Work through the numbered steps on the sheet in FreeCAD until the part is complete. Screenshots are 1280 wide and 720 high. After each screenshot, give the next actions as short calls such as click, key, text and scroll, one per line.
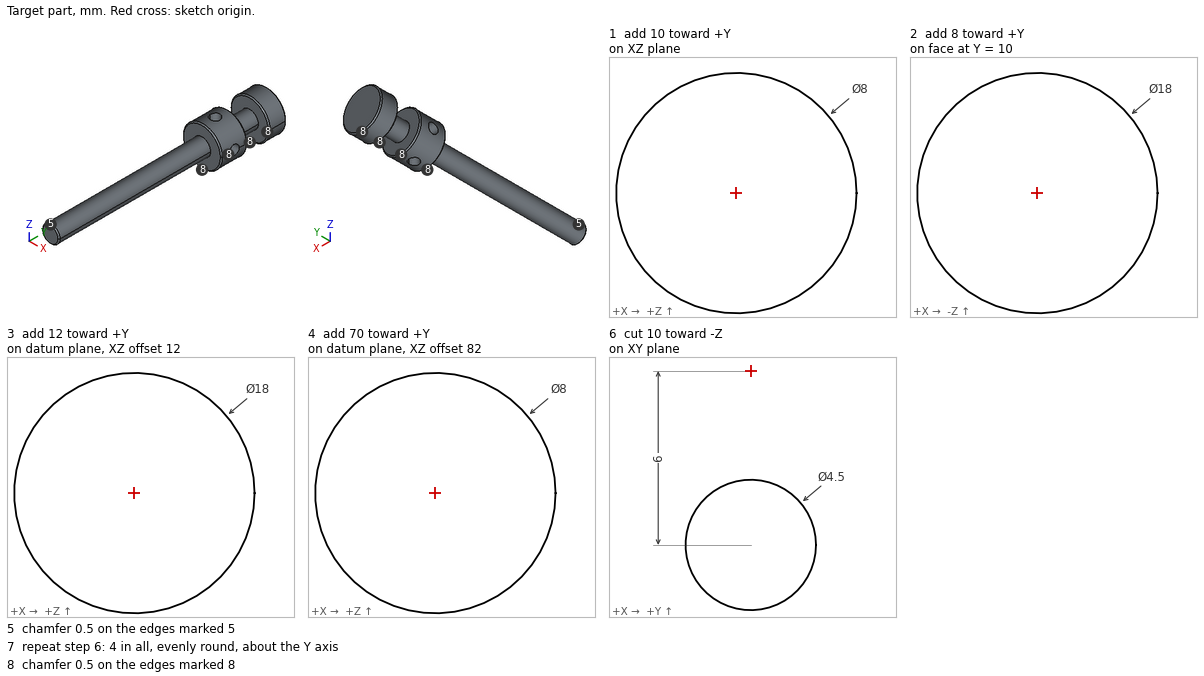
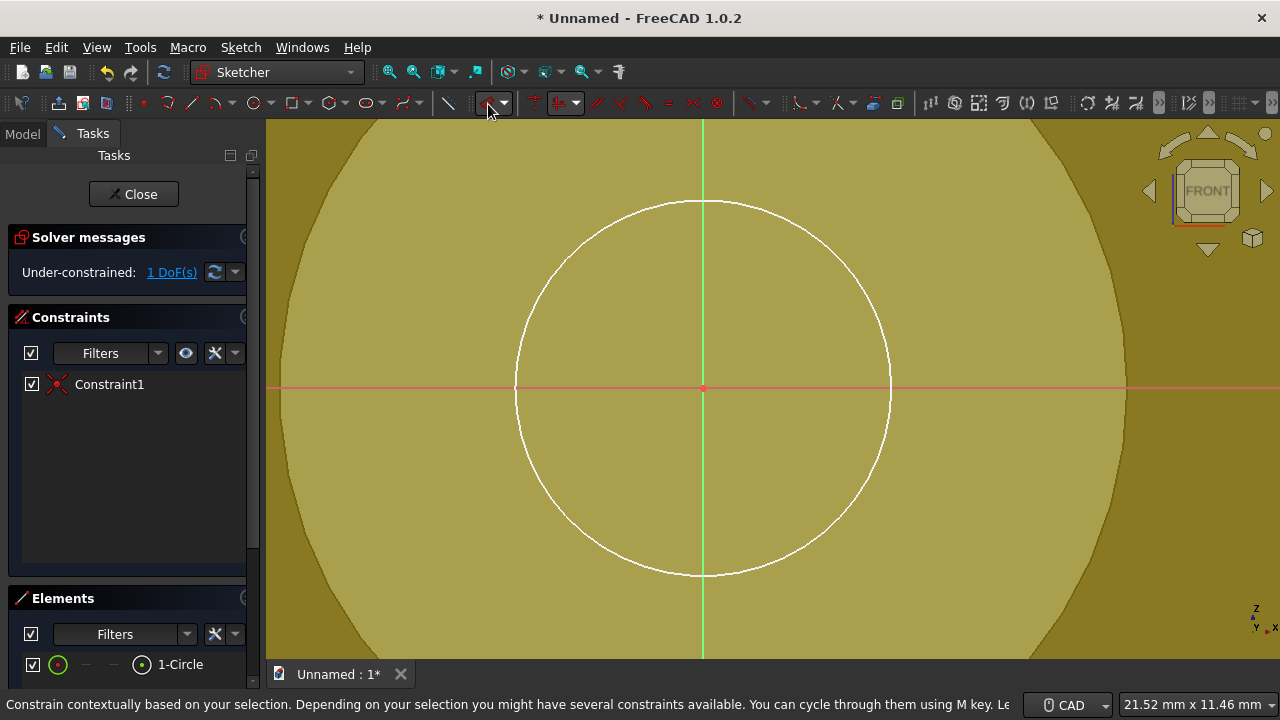
click(836, 255)
click(859, 232)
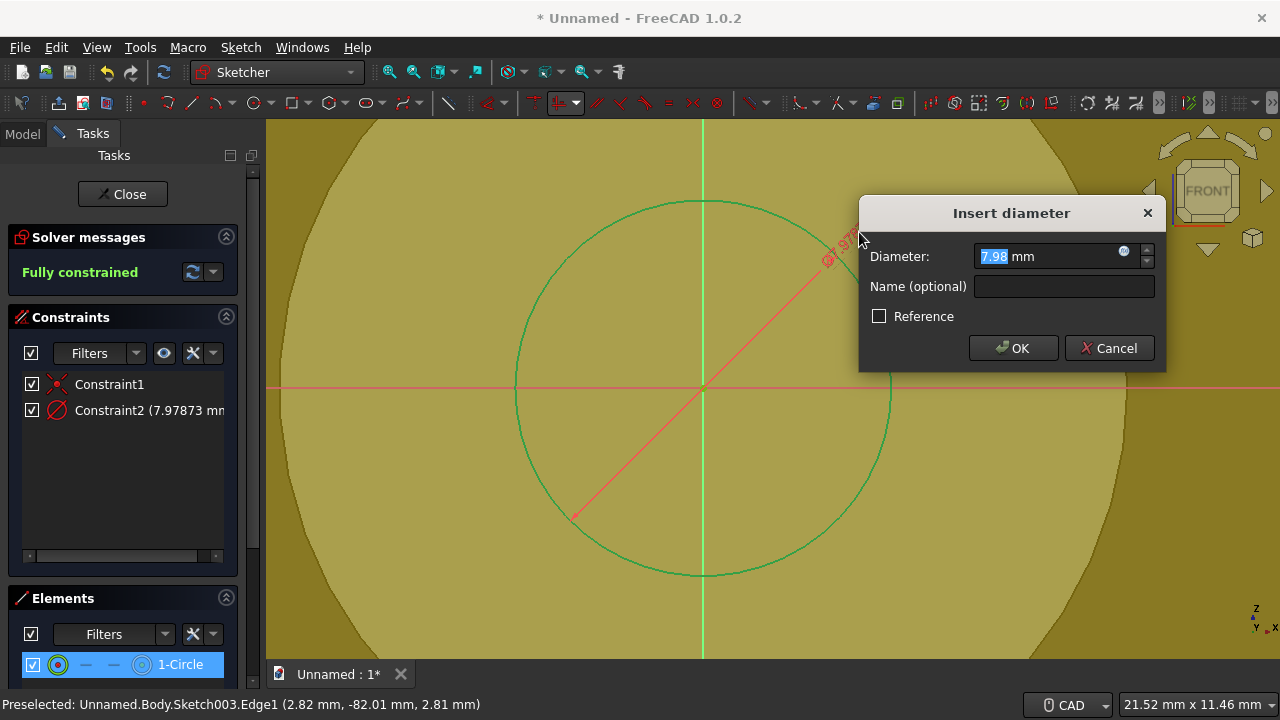
text(8)
key(Return)
key(Escape)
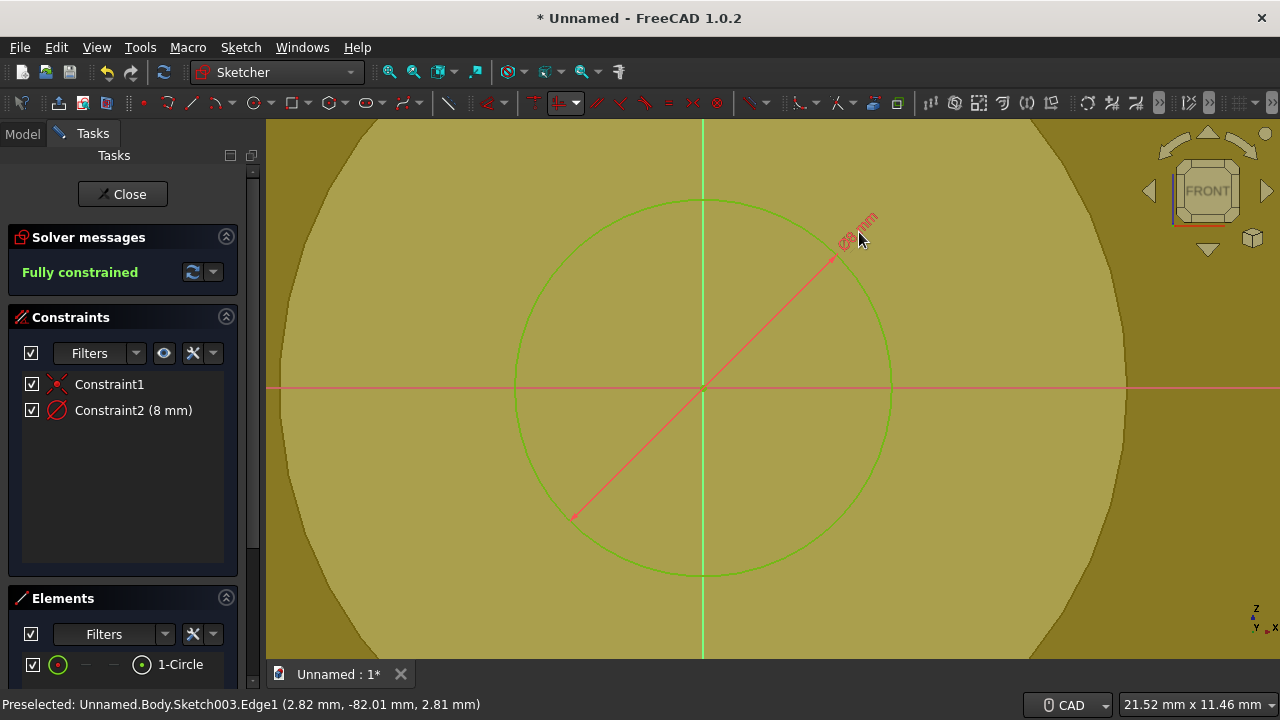
click(123, 194)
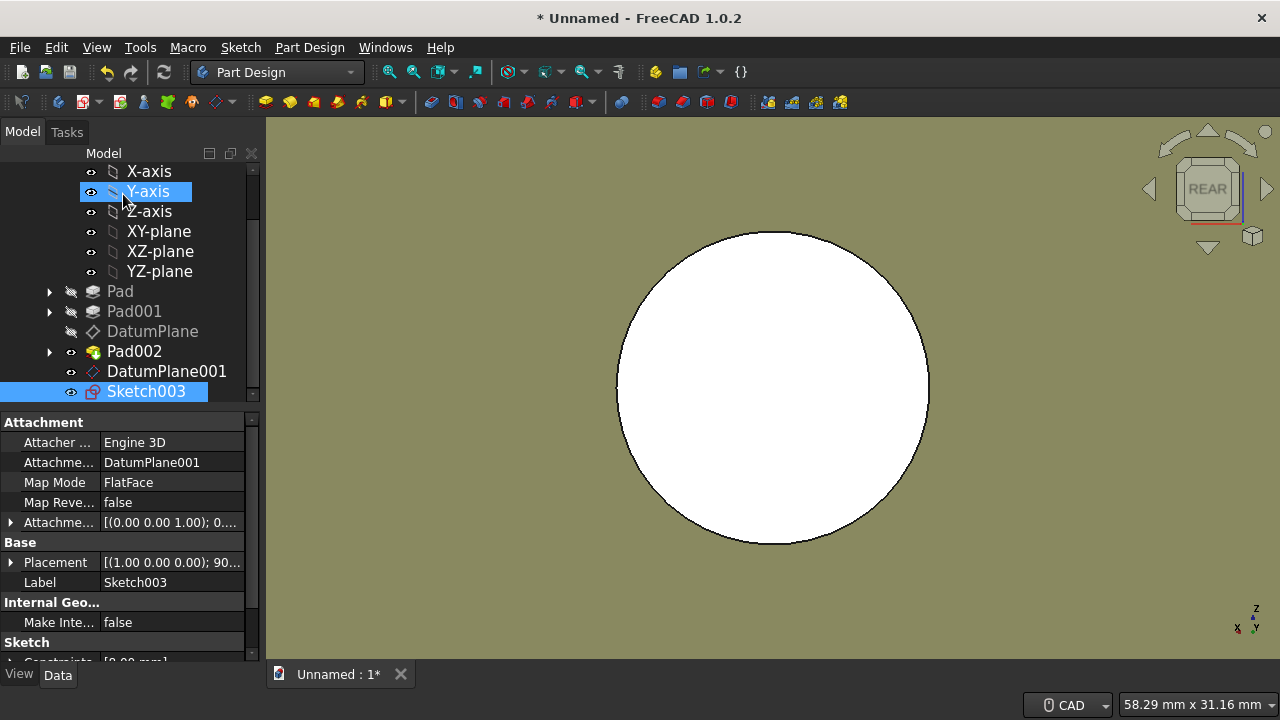
click(266, 102)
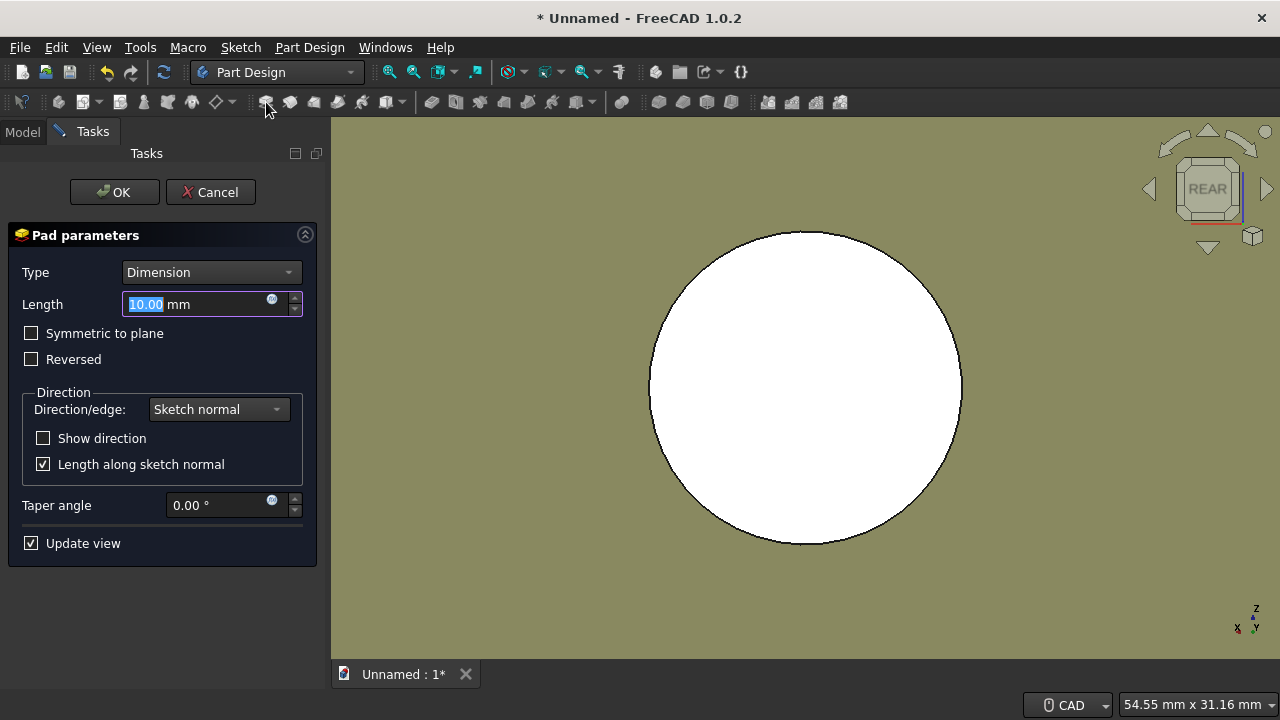
text(70)
key(Tab)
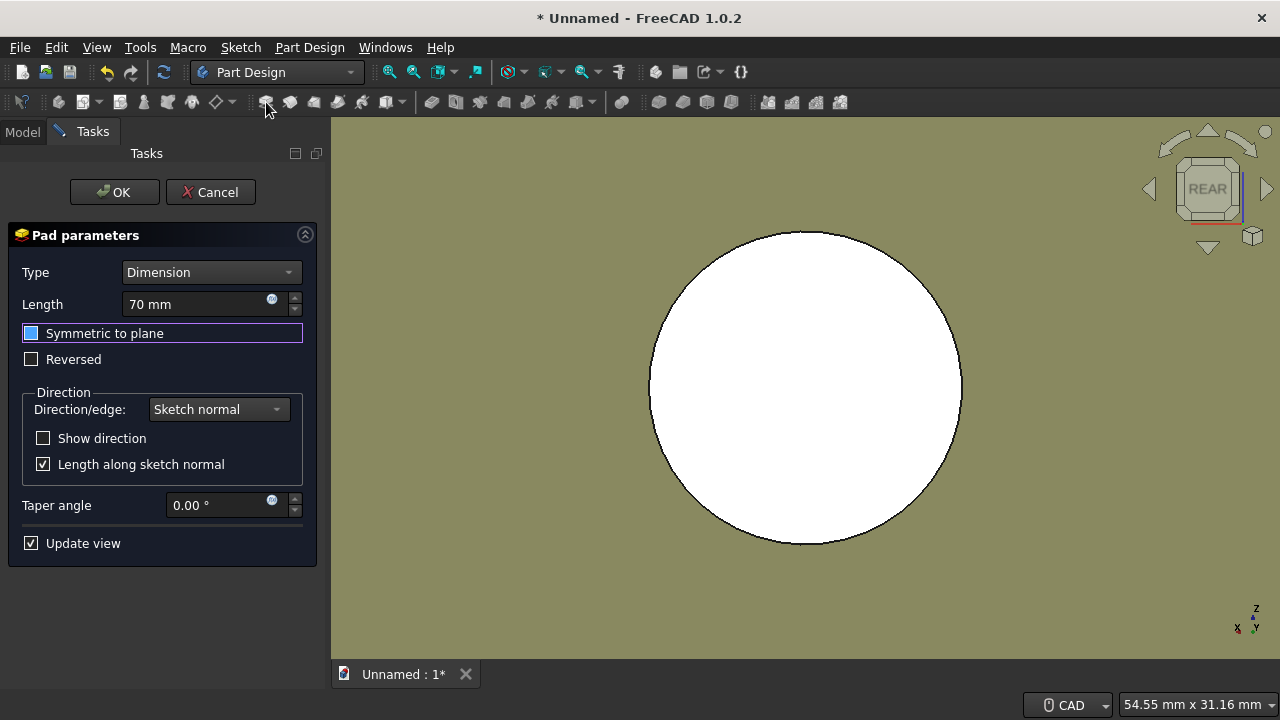
click(30, 359)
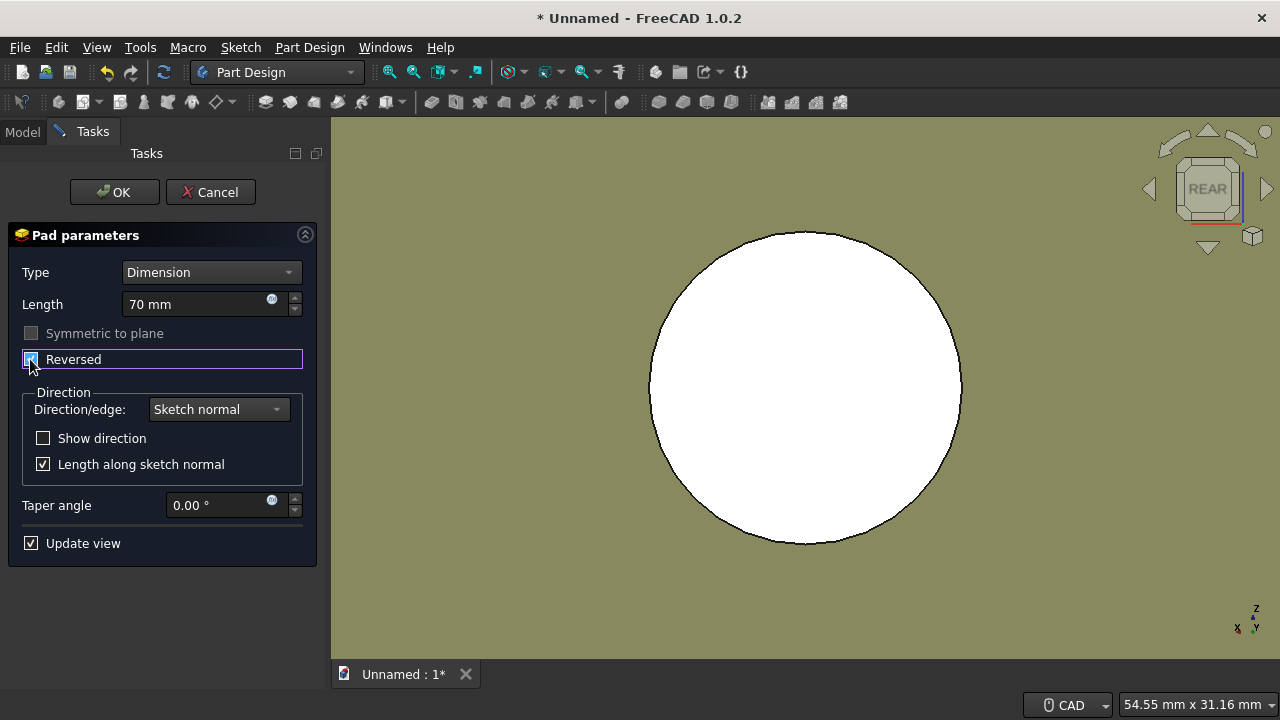
click(115, 192)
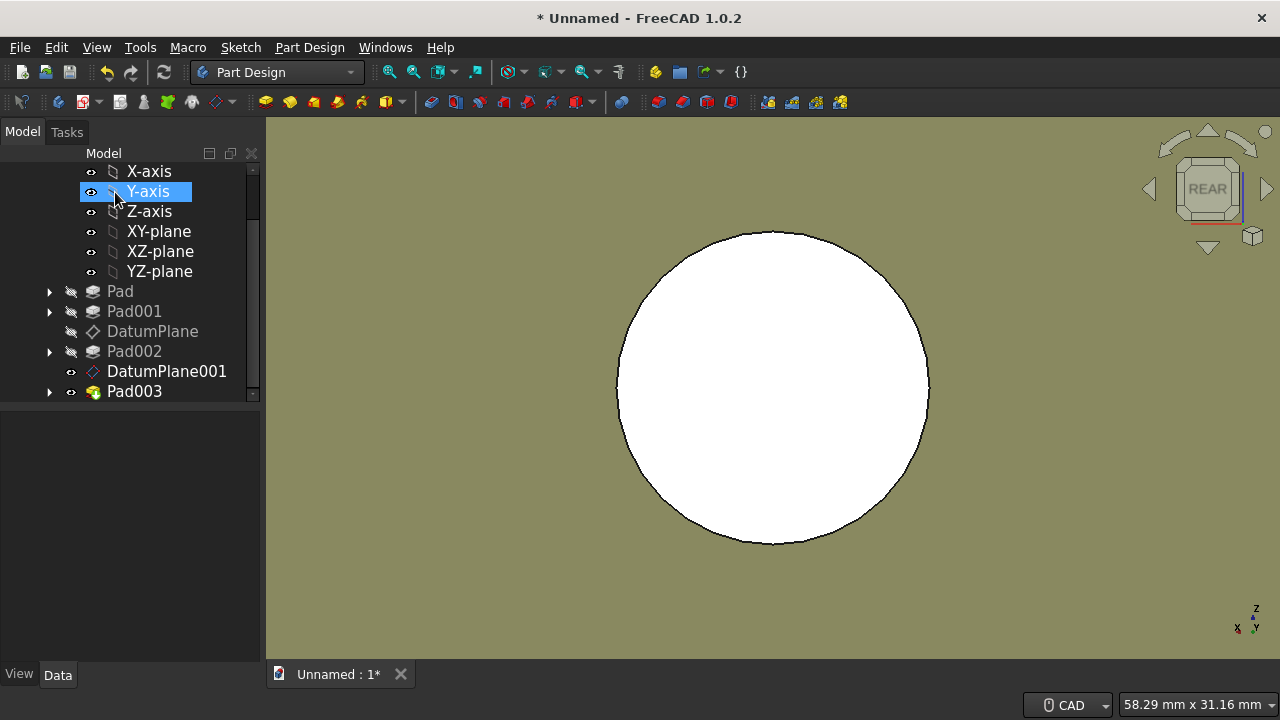
click(116, 372)
key(space)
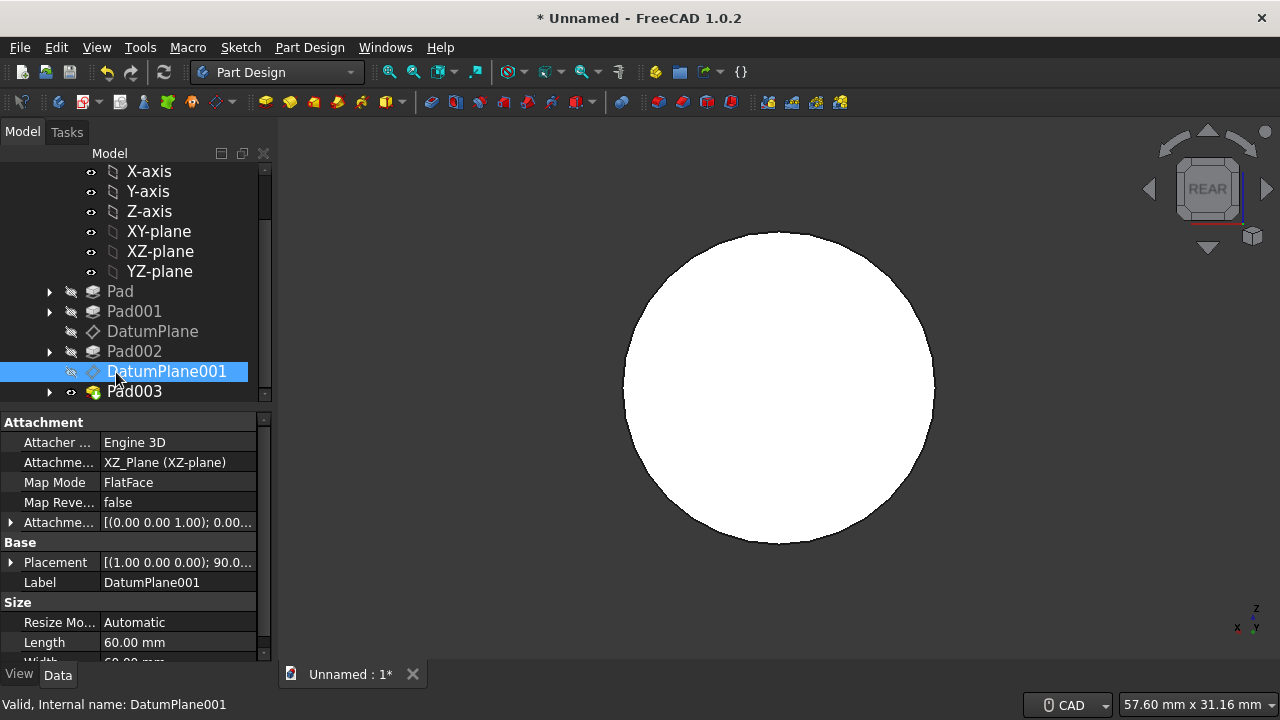
key(0)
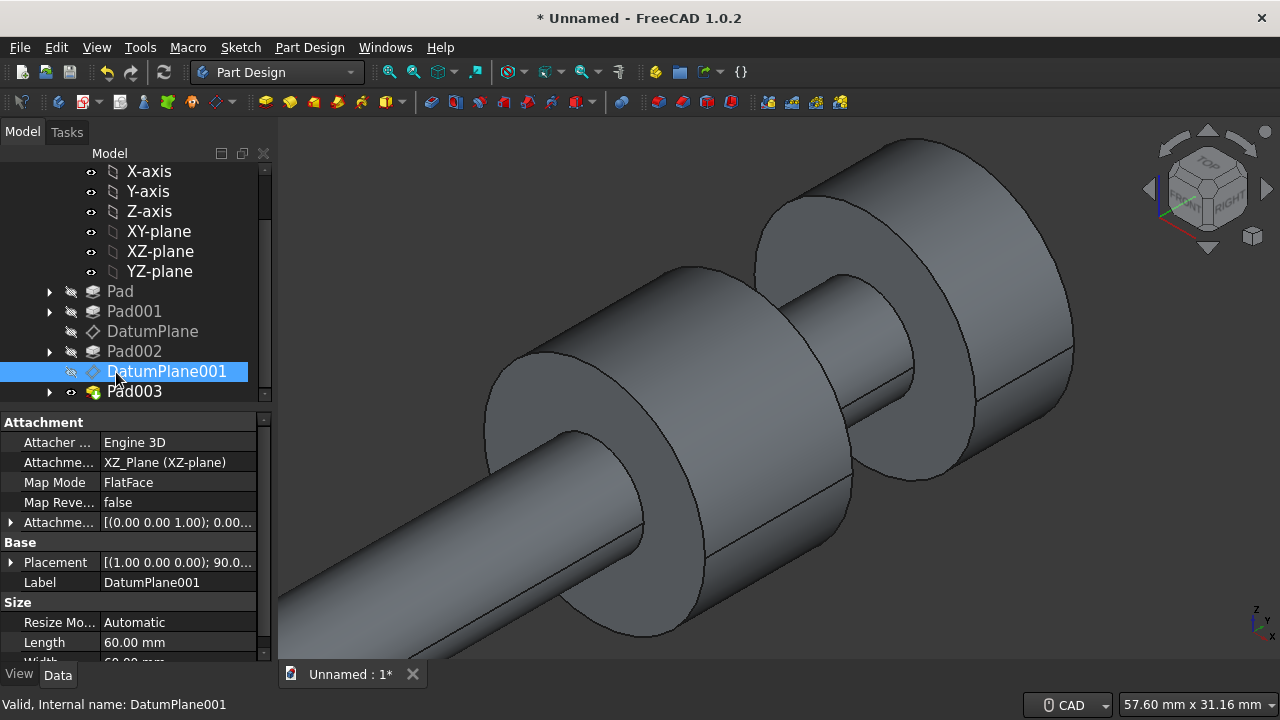
click(390, 72)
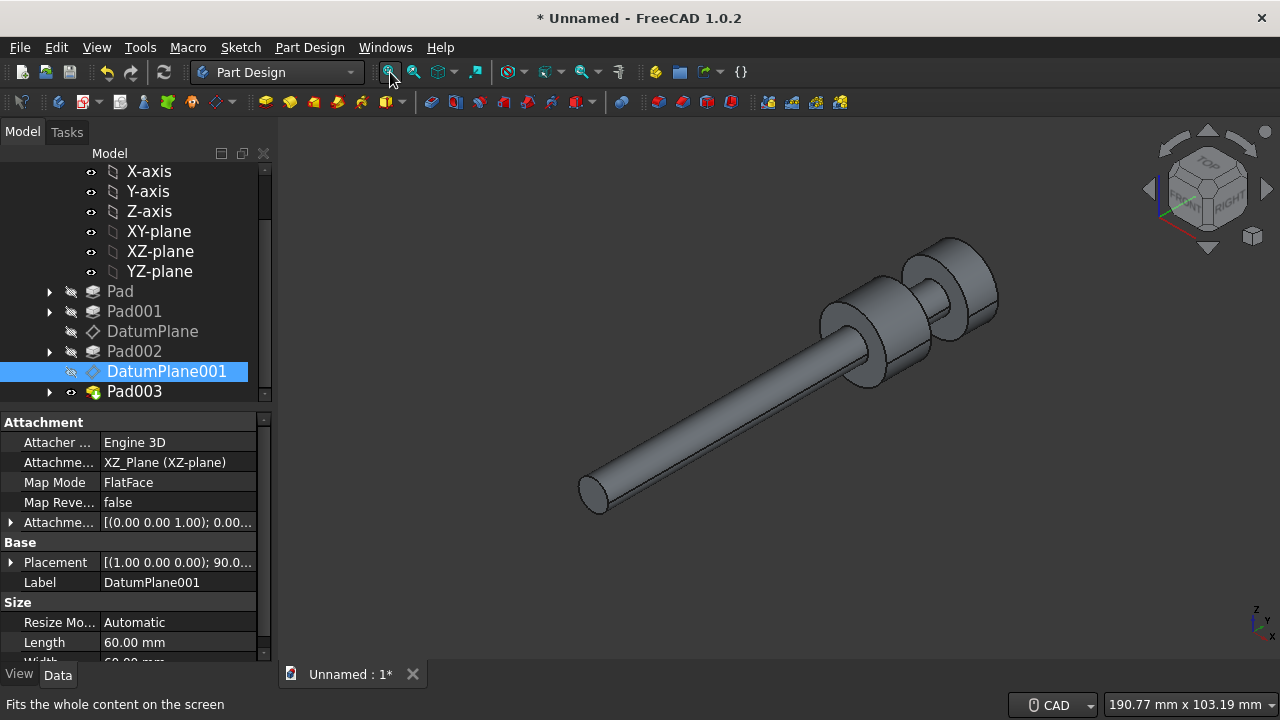
click(578, 486)